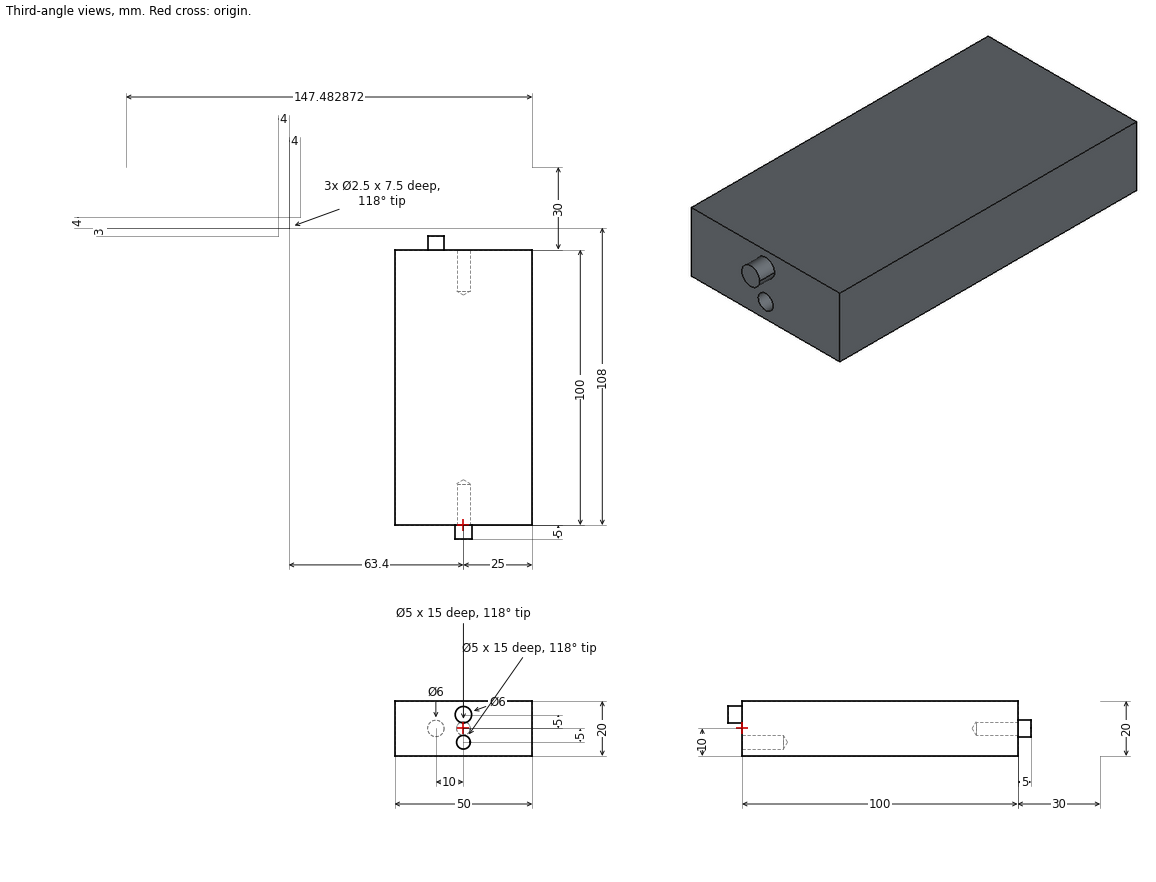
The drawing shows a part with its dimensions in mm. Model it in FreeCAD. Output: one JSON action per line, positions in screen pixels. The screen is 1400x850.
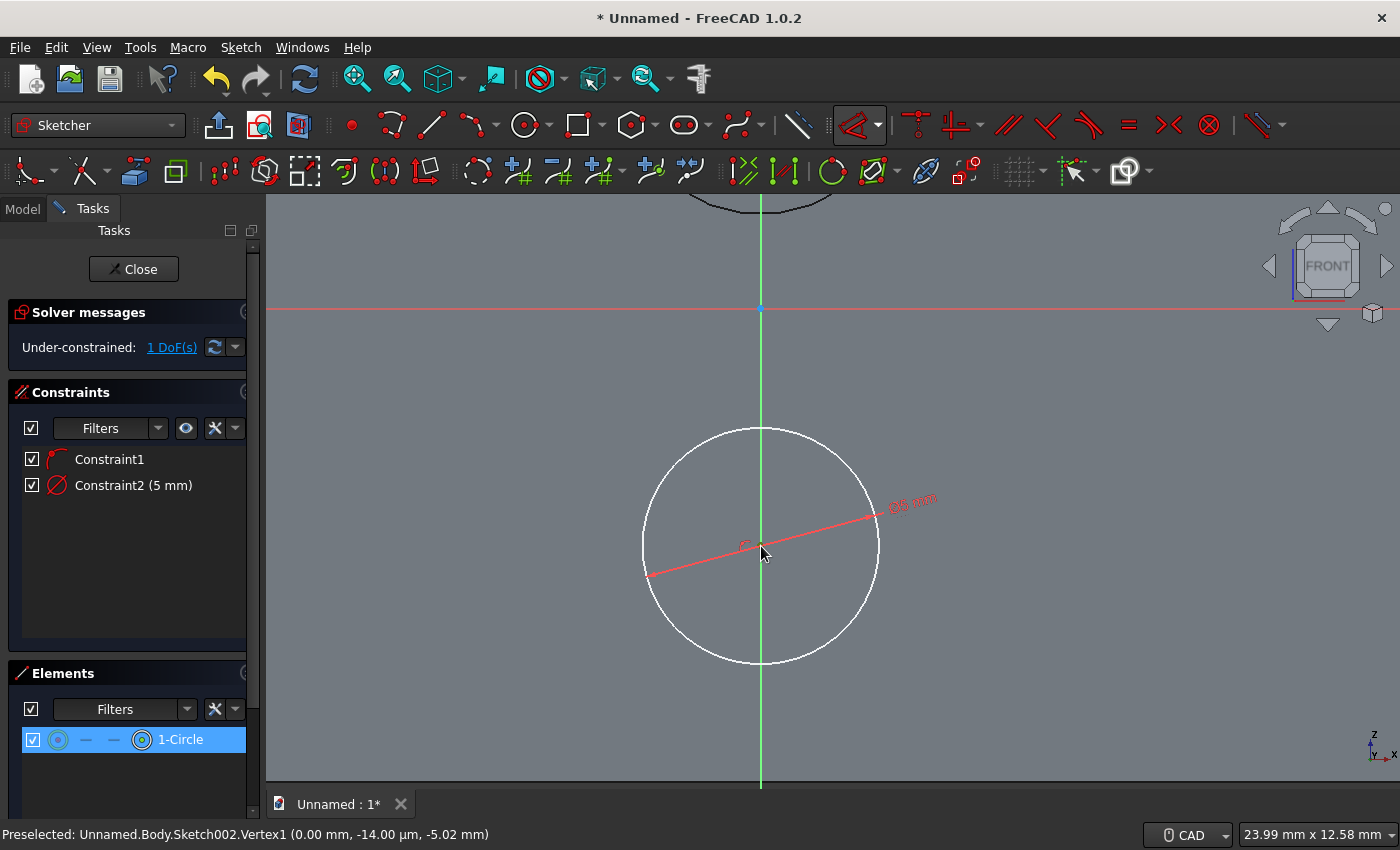
{"action": "key", "text": "i"}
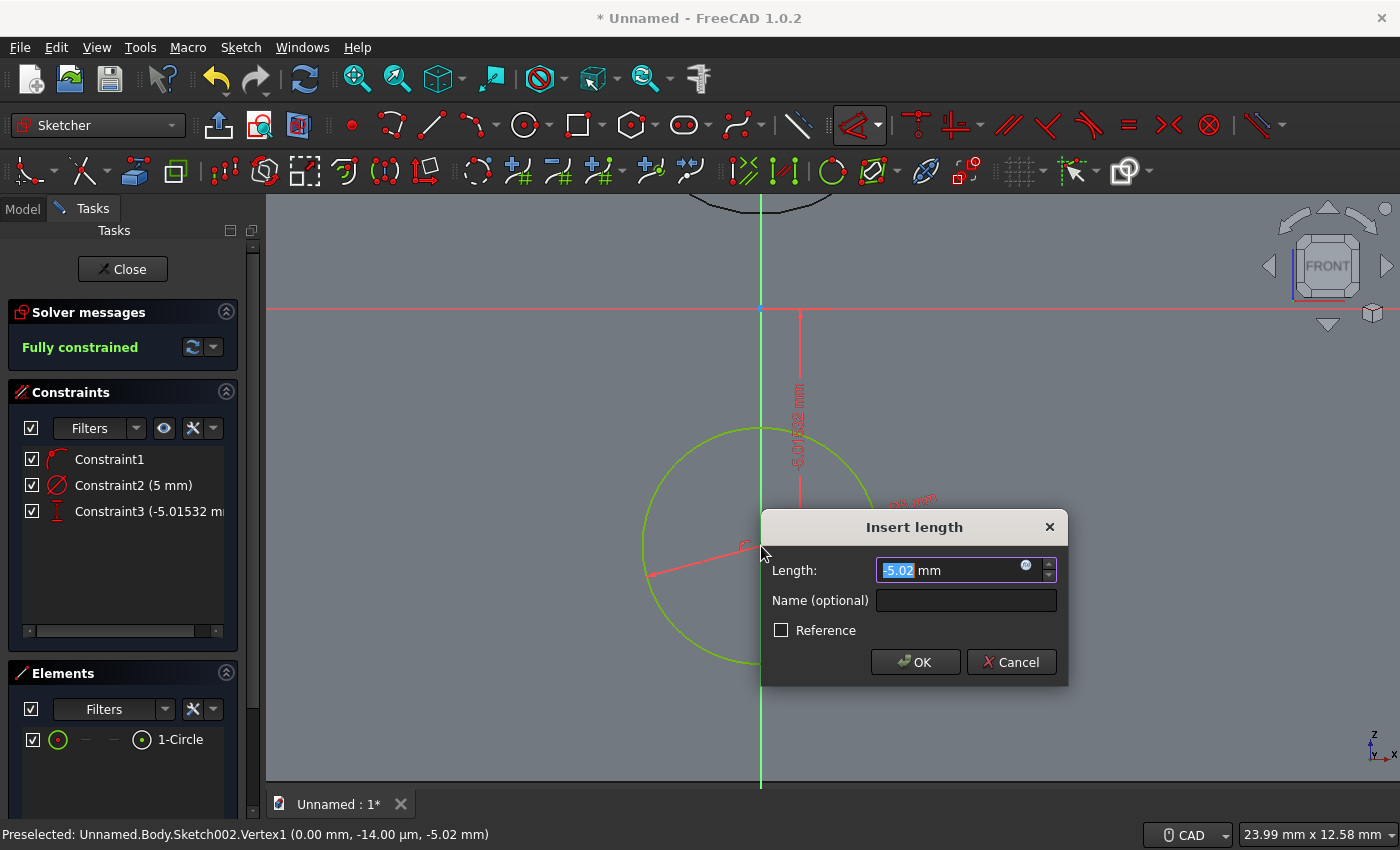
{"action": "type", "text": "-5"}
{"action": "key", "text": "Return"}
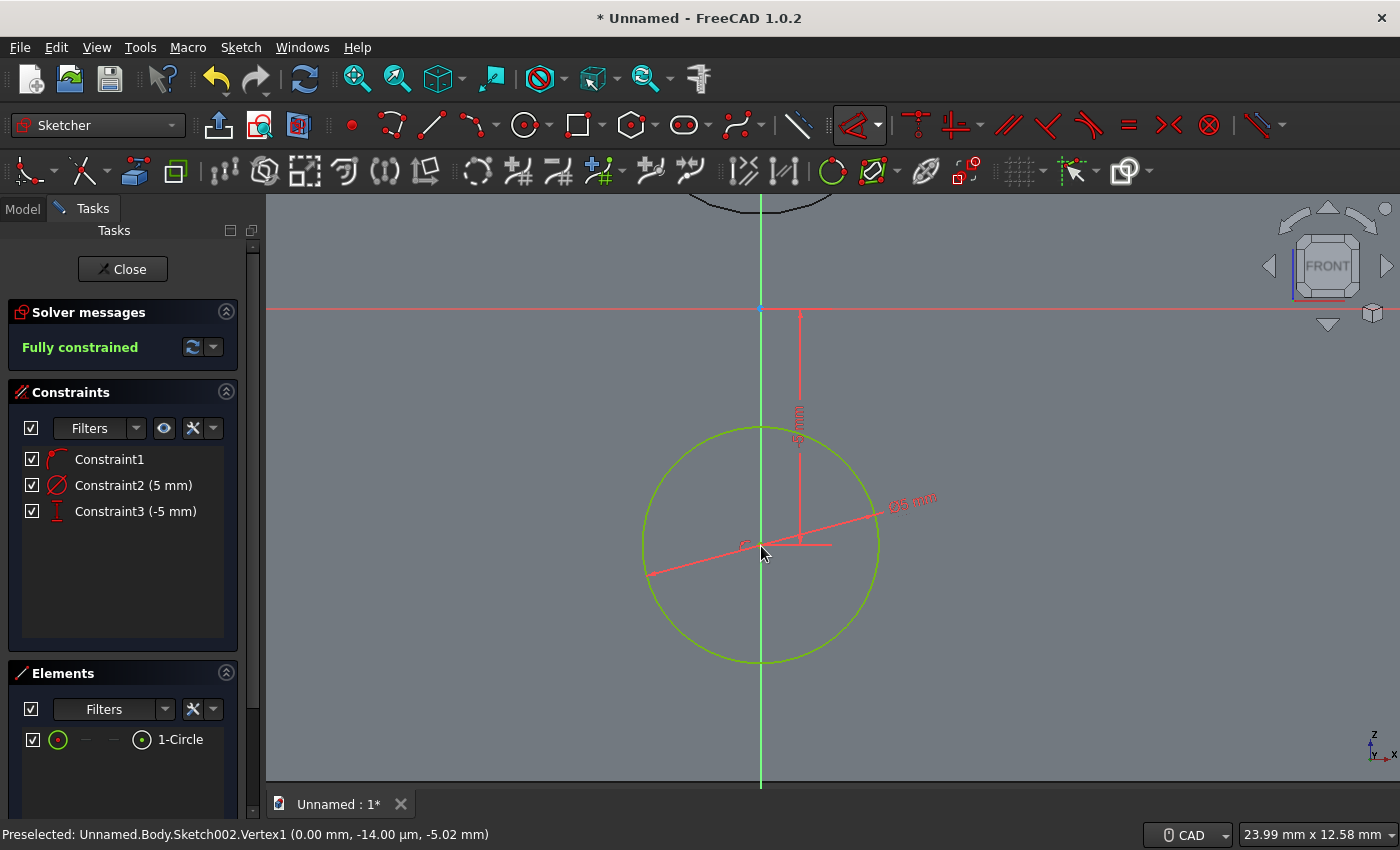
{"action": "left_click", "coordinate": [123, 269]}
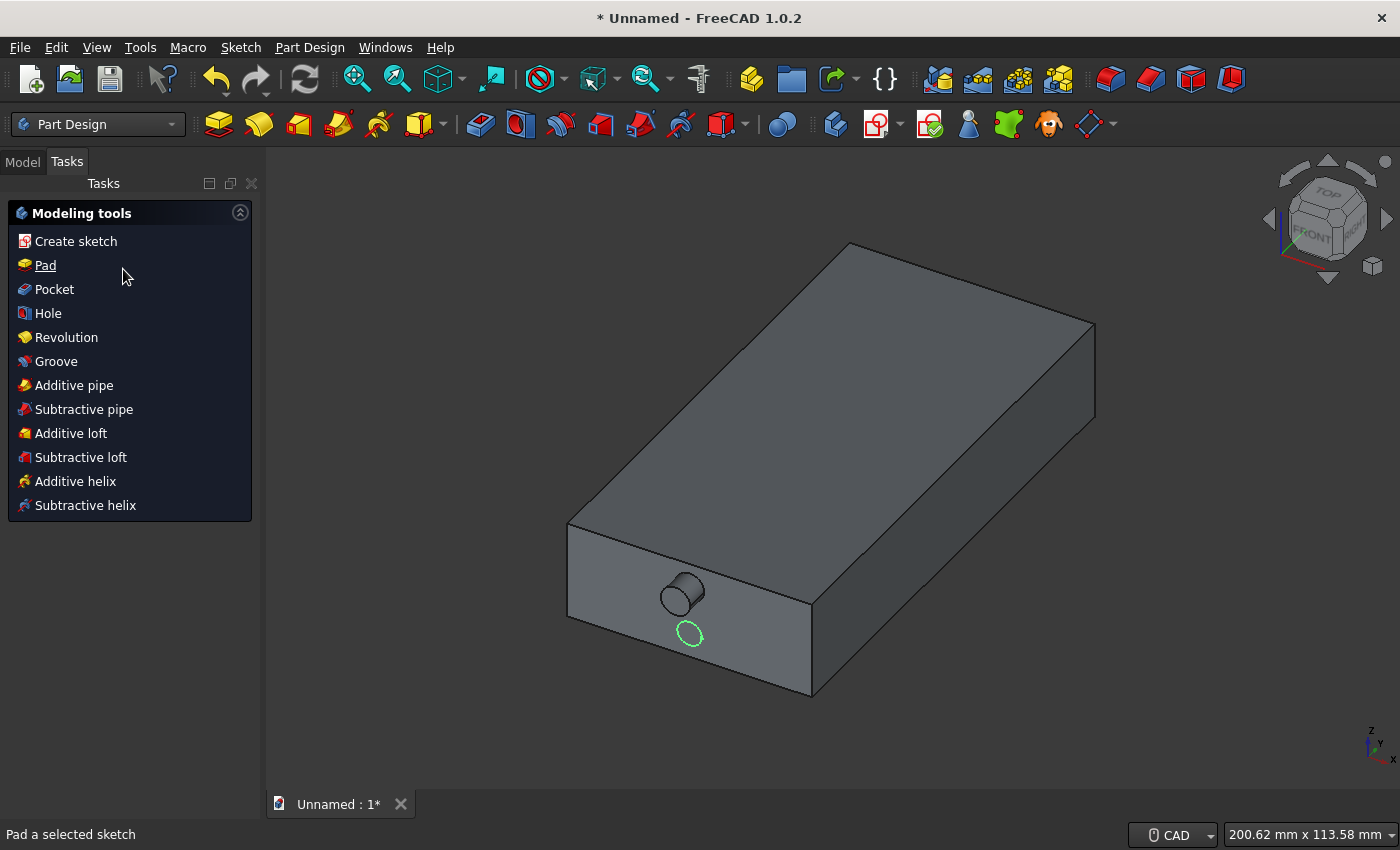
{"action": "left_click", "coordinate": [522, 124]}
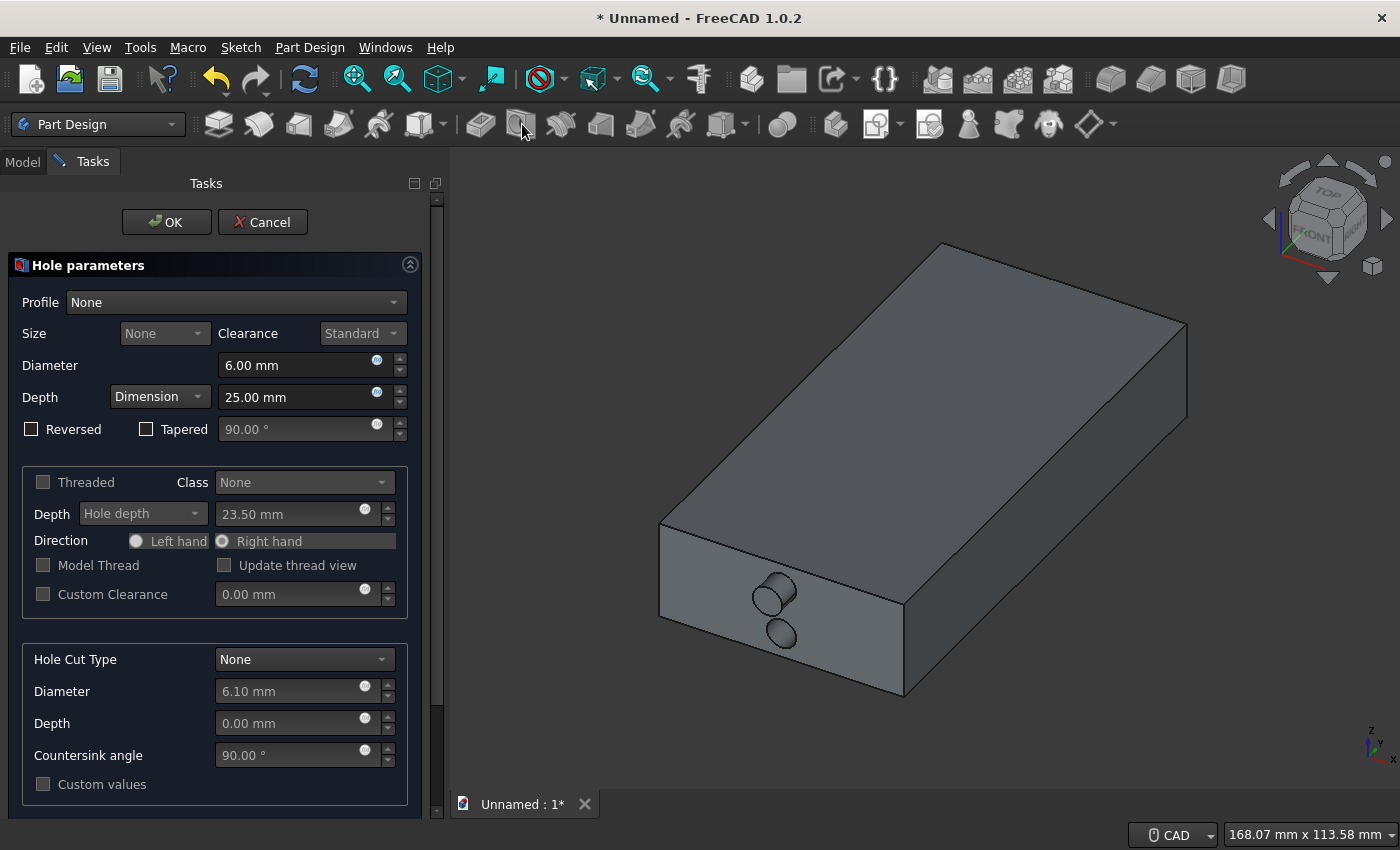
{"action": "triple_click", "coordinate": [305, 365]}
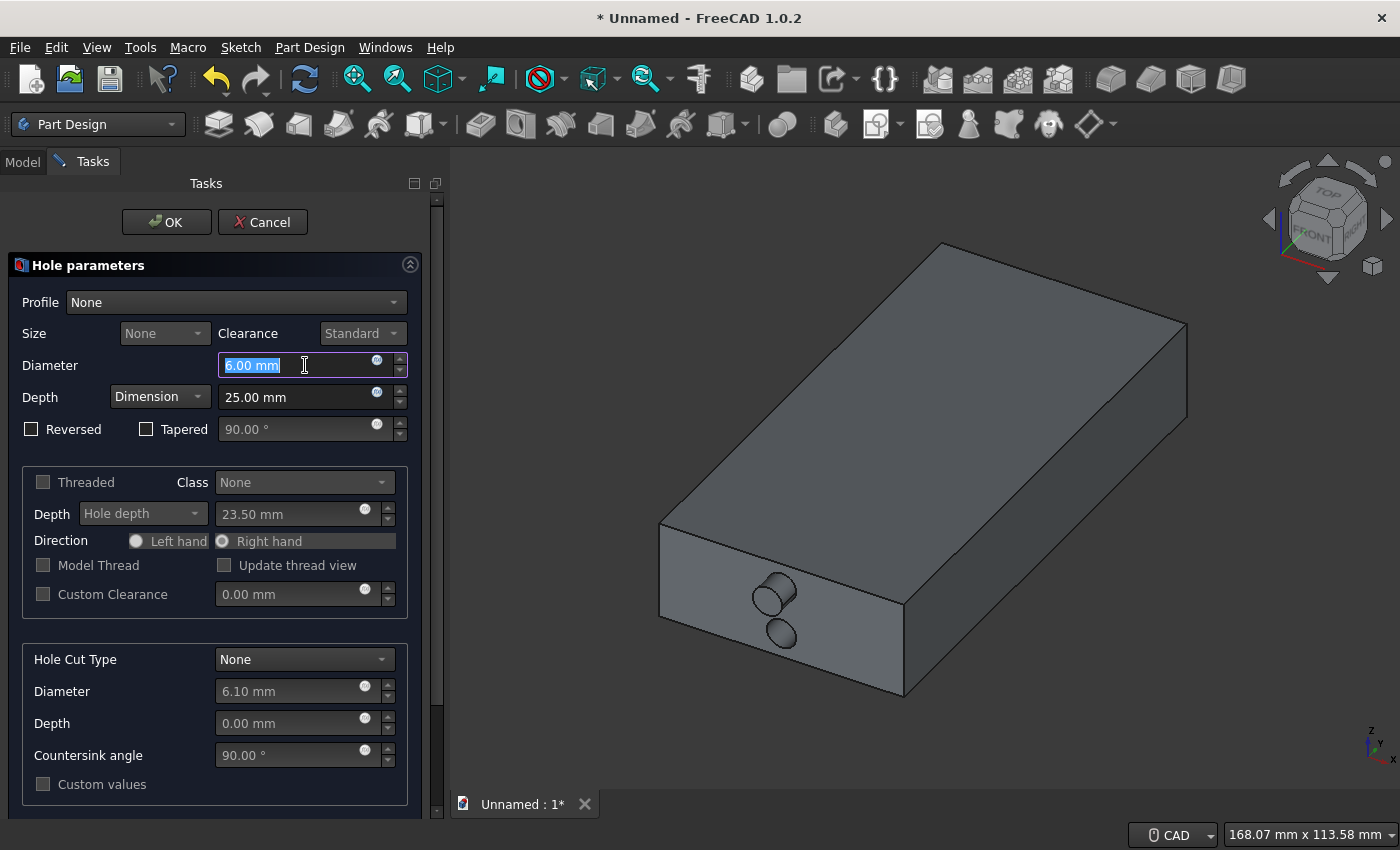
{"action": "type", "text": "5"}
{"action": "key", "text": "Tab"}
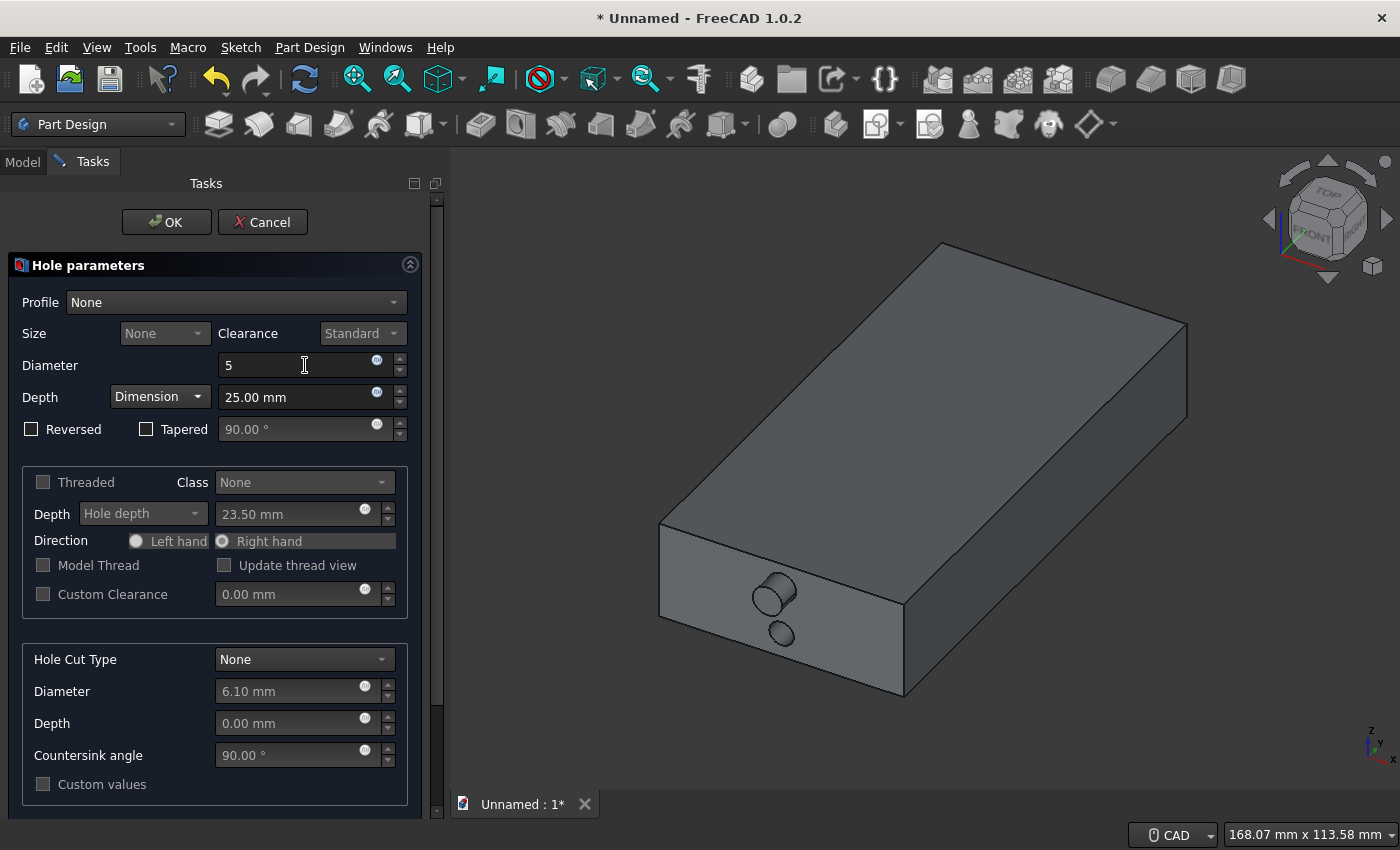
{"action": "triple_click", "coordinate": [305, 397]}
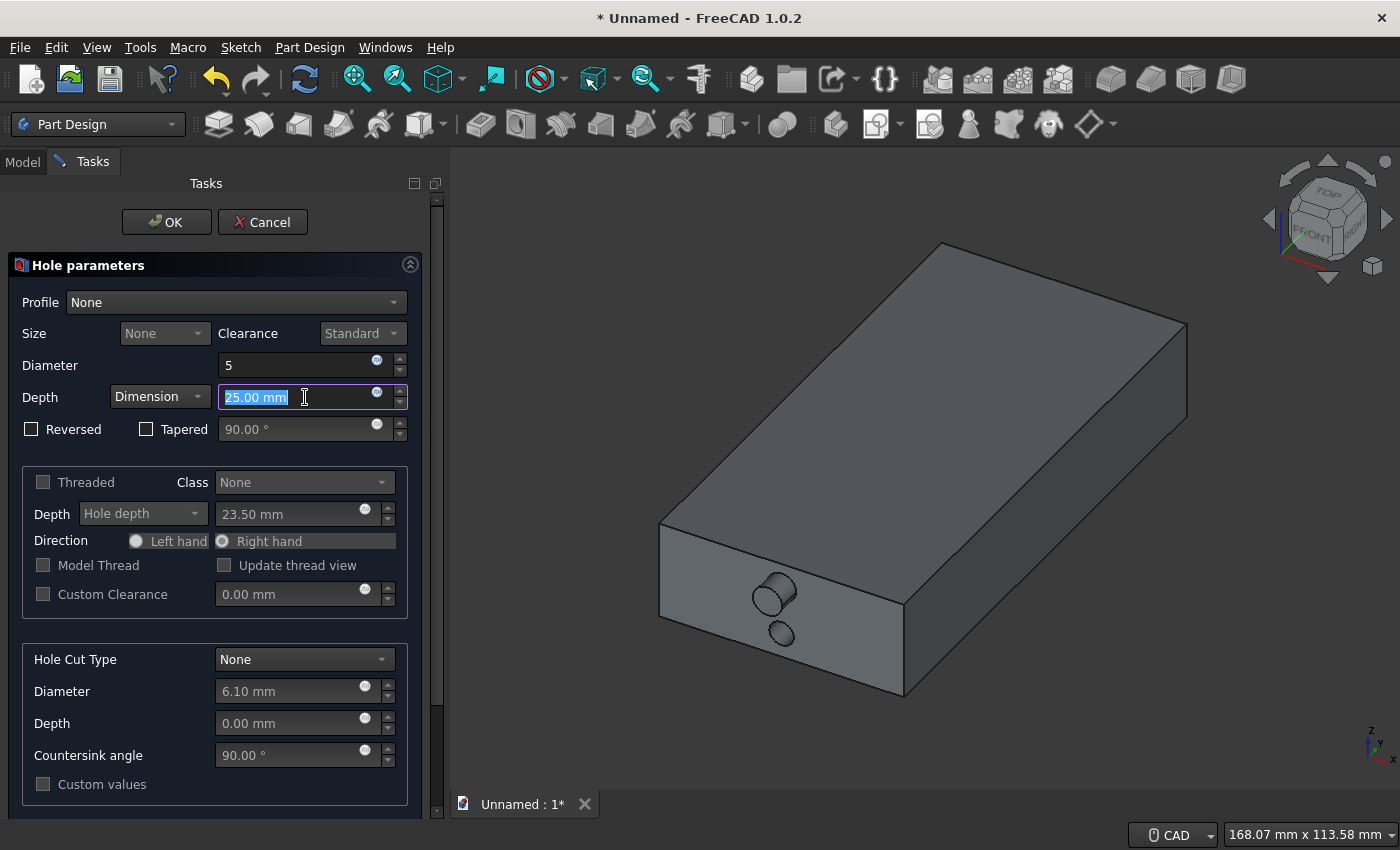
{"action": "type", "text": "15"}
{"action": "key", "text": "Tab"}